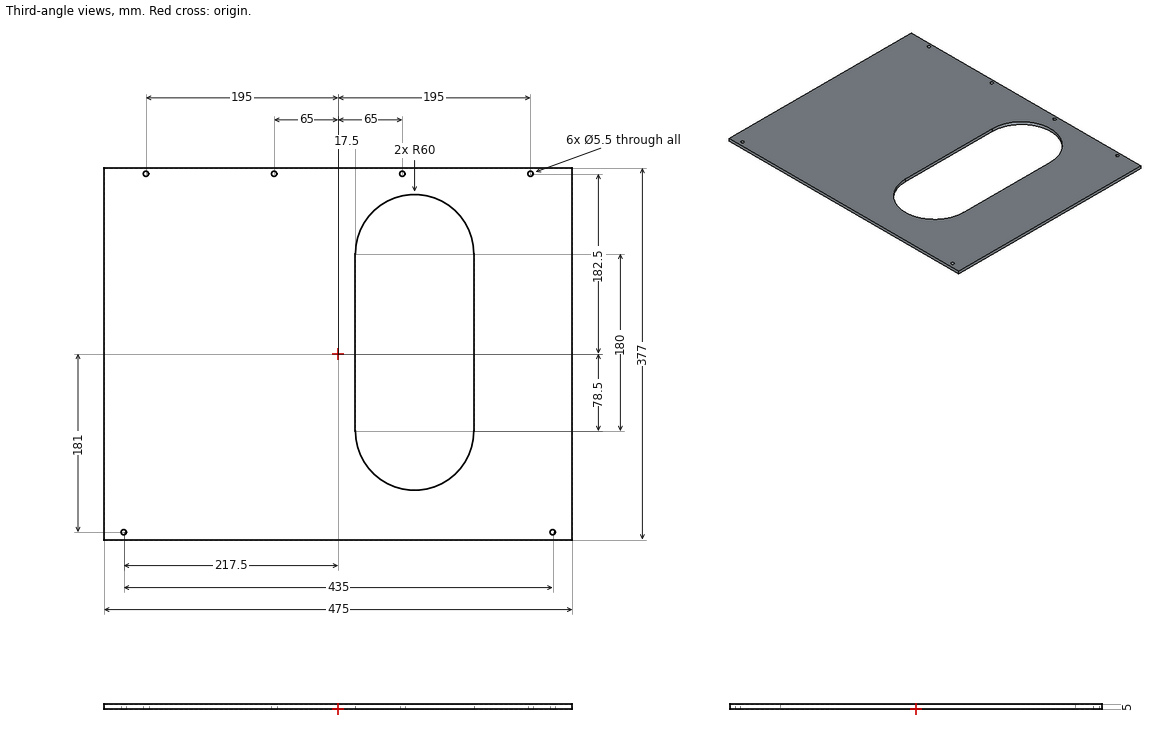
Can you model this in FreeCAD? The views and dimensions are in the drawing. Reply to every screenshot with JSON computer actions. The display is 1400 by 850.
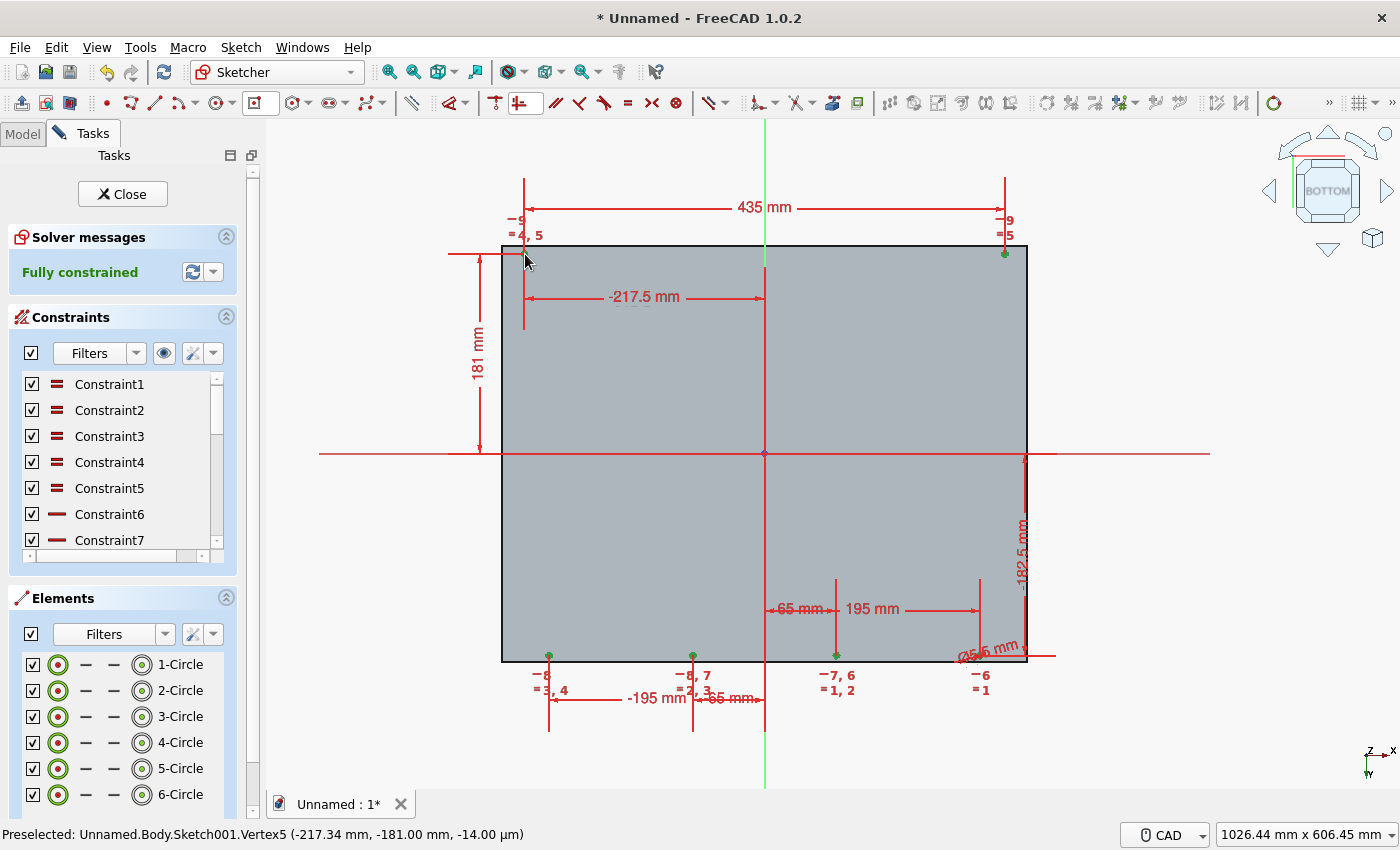
{"action": "left_click", "coordinate": [123, 194]}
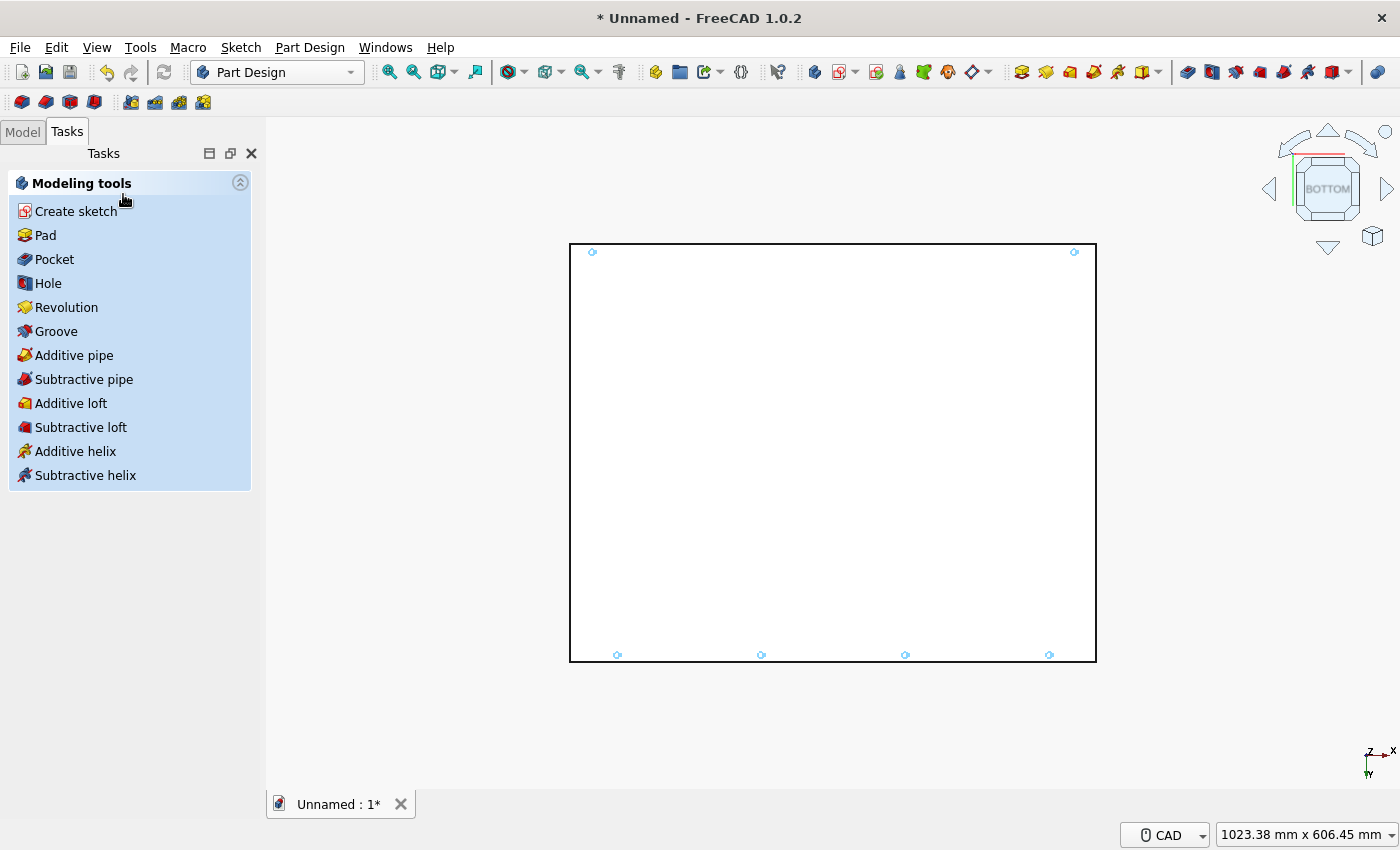
{"action": "left_click", "coordinate": [1212, 72]}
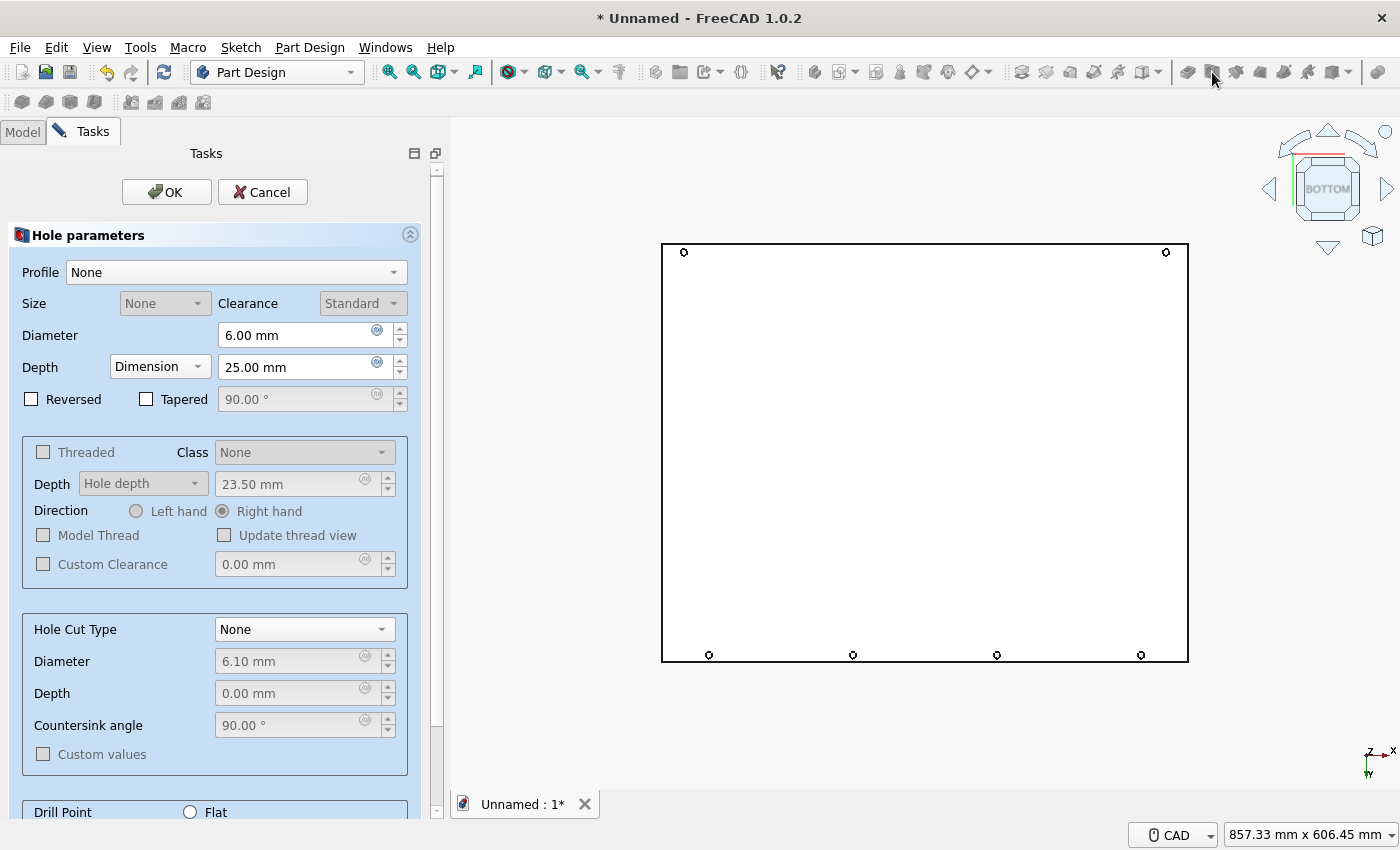
{"action": "triple_click", "coordinate": [305, 335]}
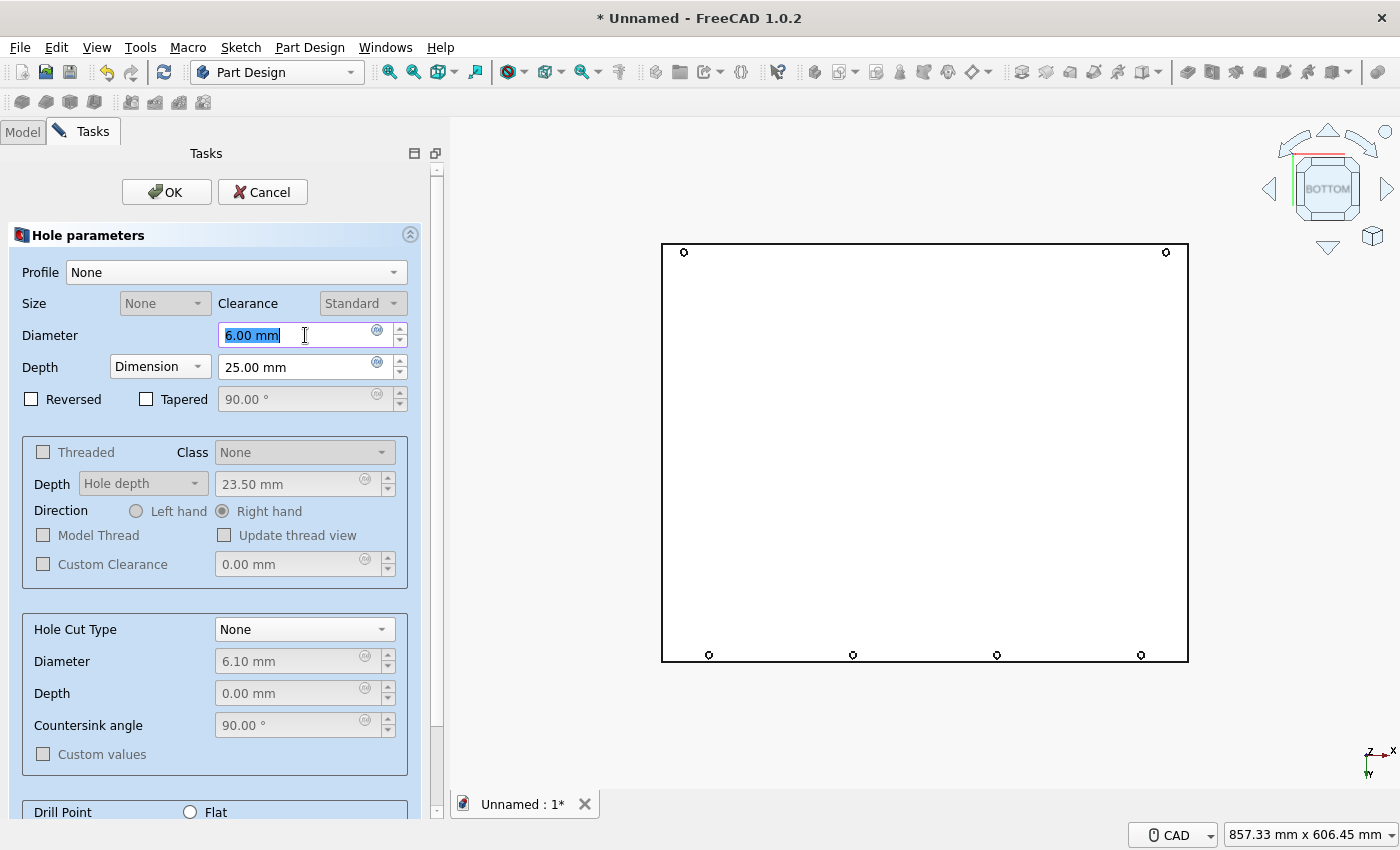
{"action": "type", "text": "5.5"}
{"action": "key", "text": "Tab"}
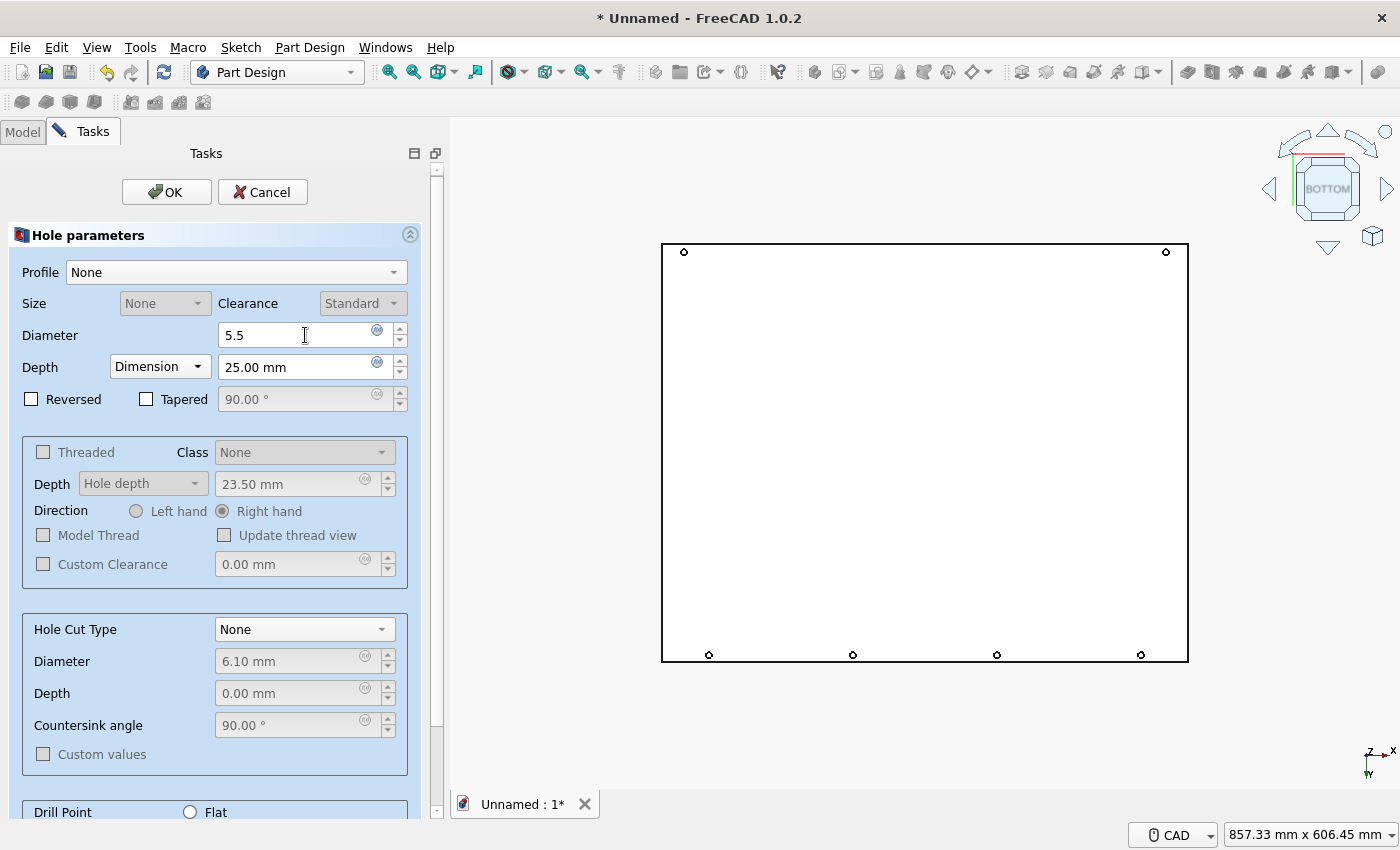
{"action": "left_click", "coordinate": [161, 366]}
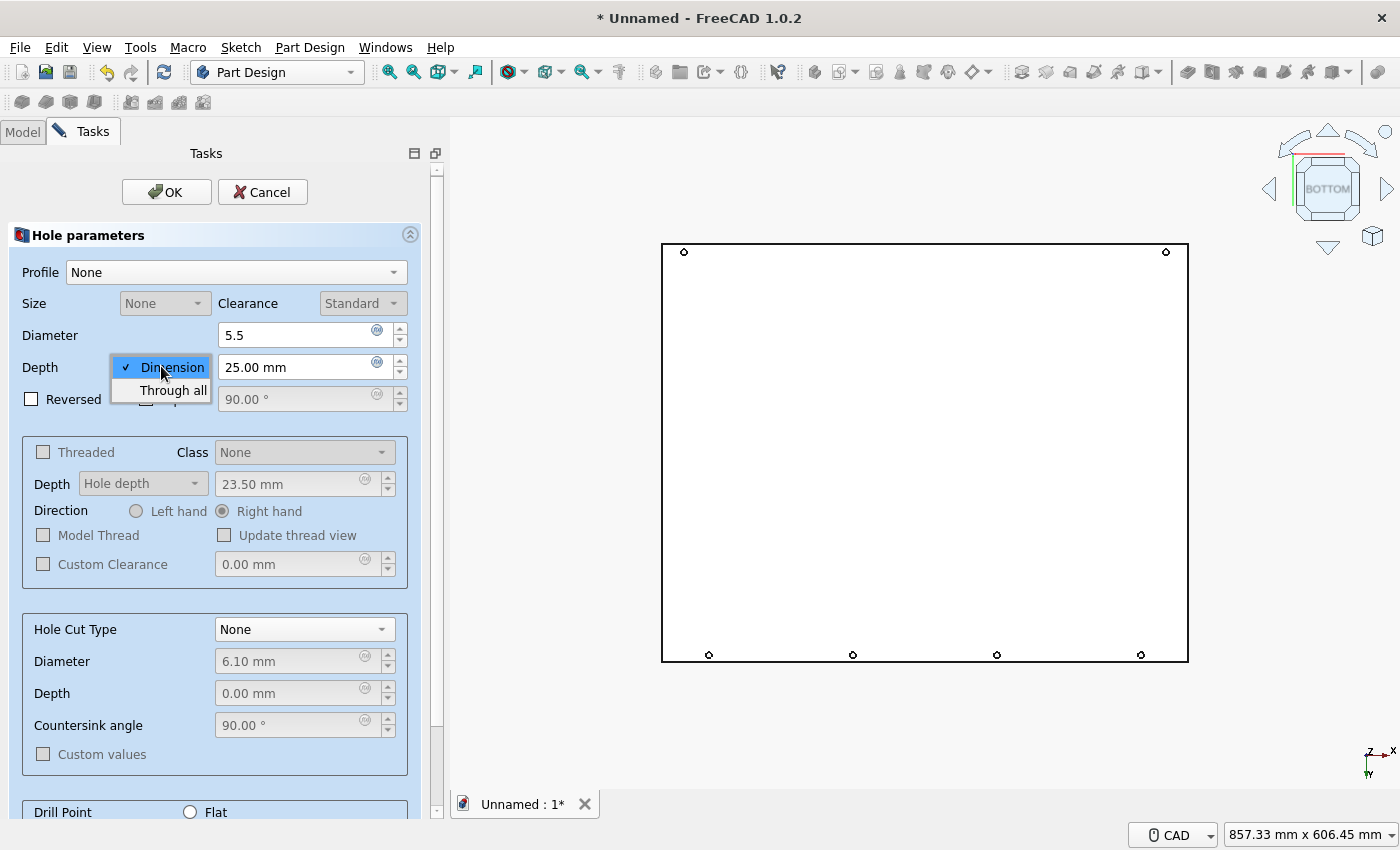
{"action": "left_click", "coordinate": [160, 390]}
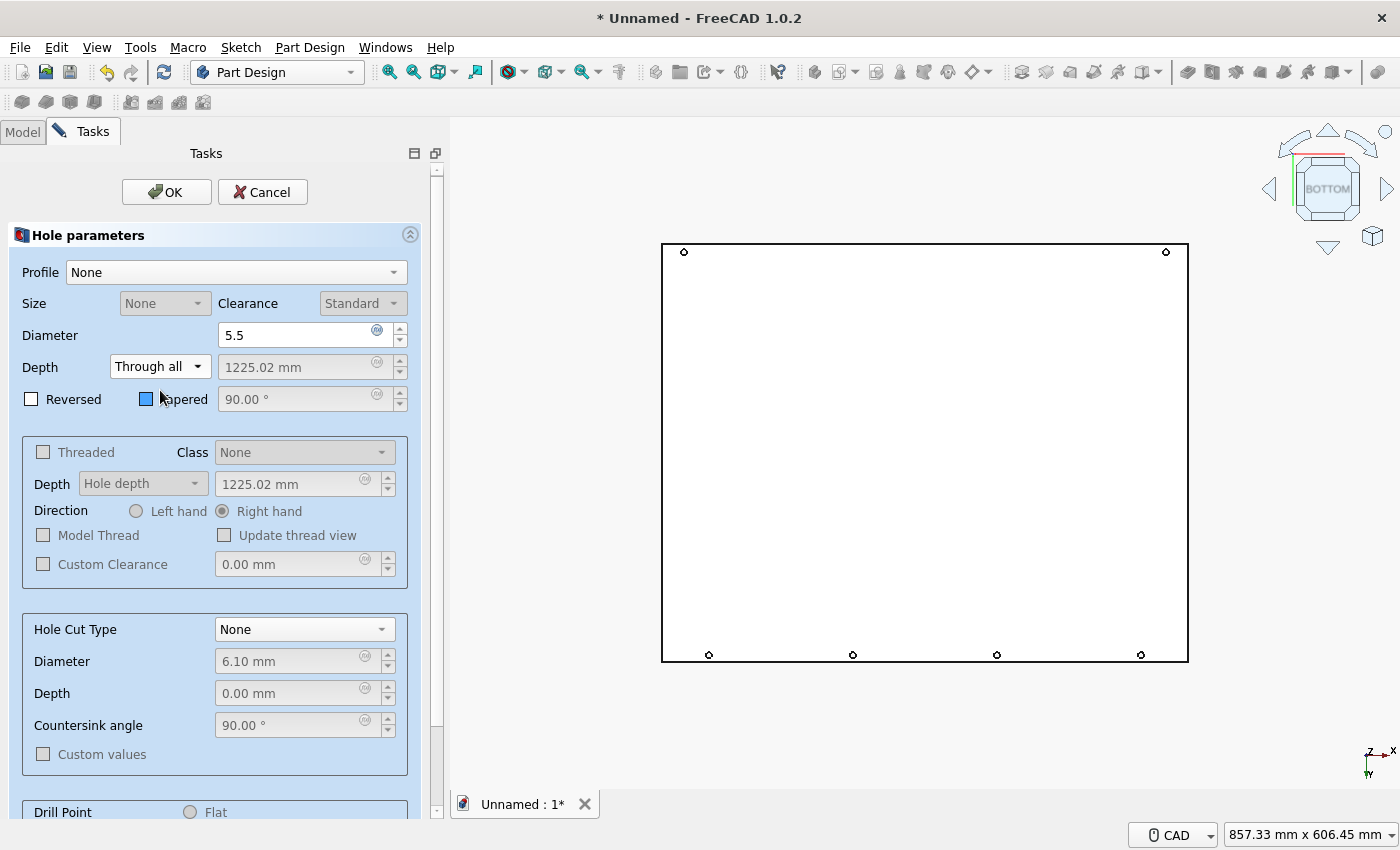
{"action": "left_click", "coordinate": [167, 192]}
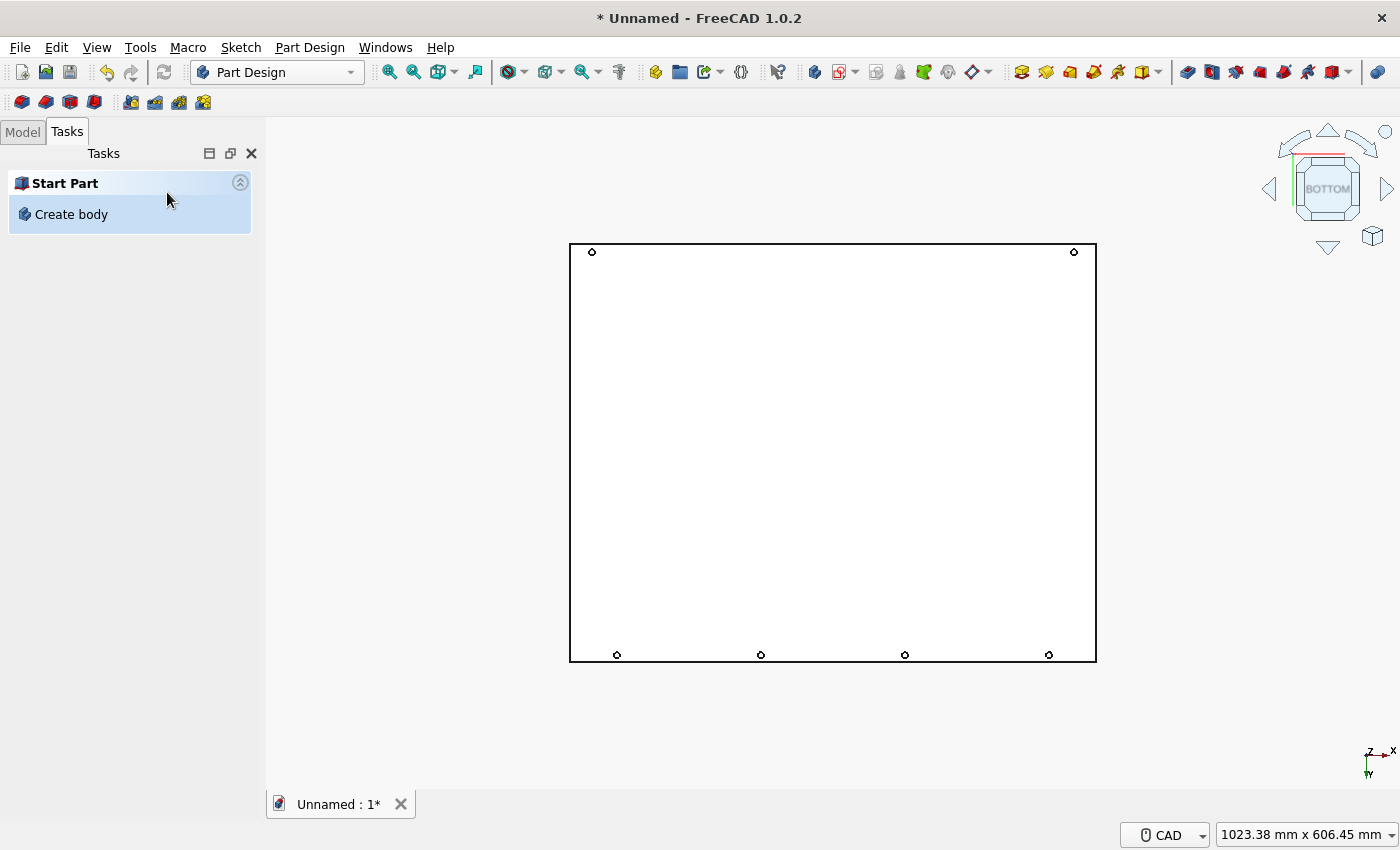
{"action": "left_click", "coordinate": [833, 452]}